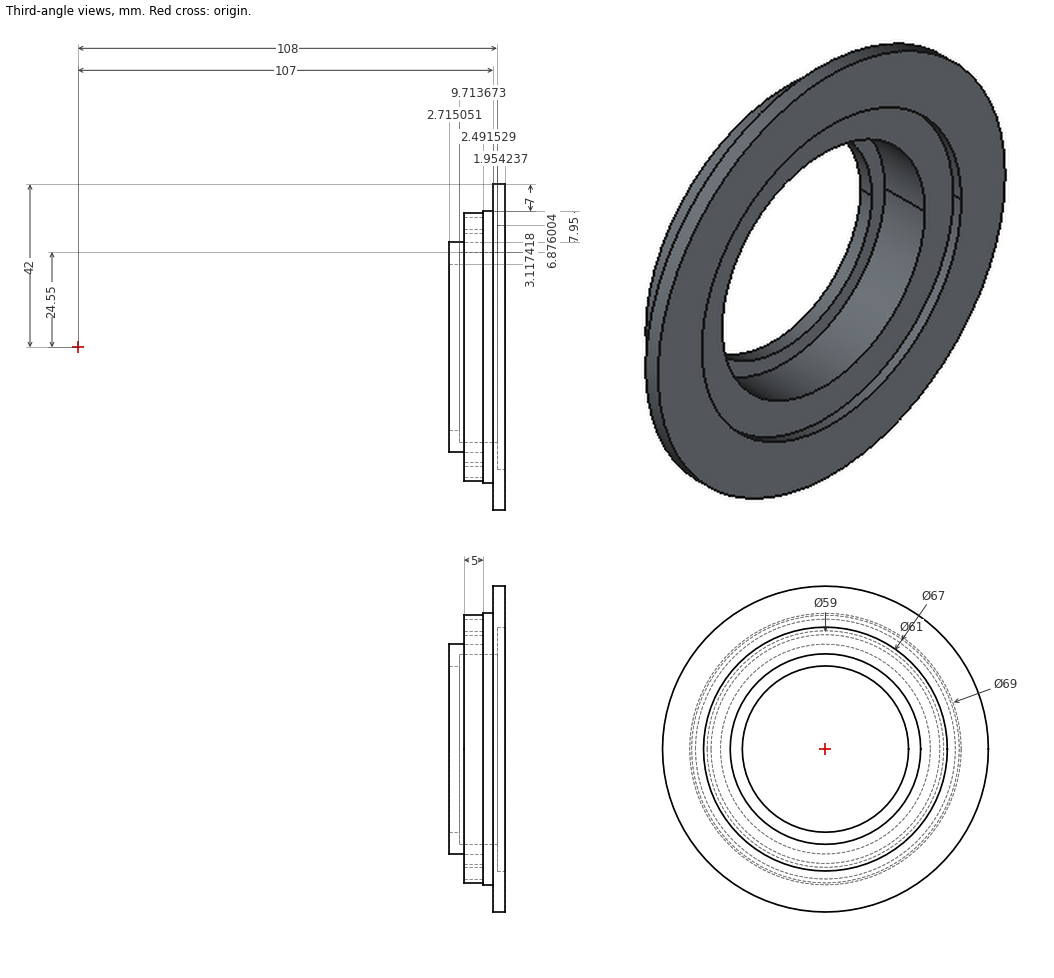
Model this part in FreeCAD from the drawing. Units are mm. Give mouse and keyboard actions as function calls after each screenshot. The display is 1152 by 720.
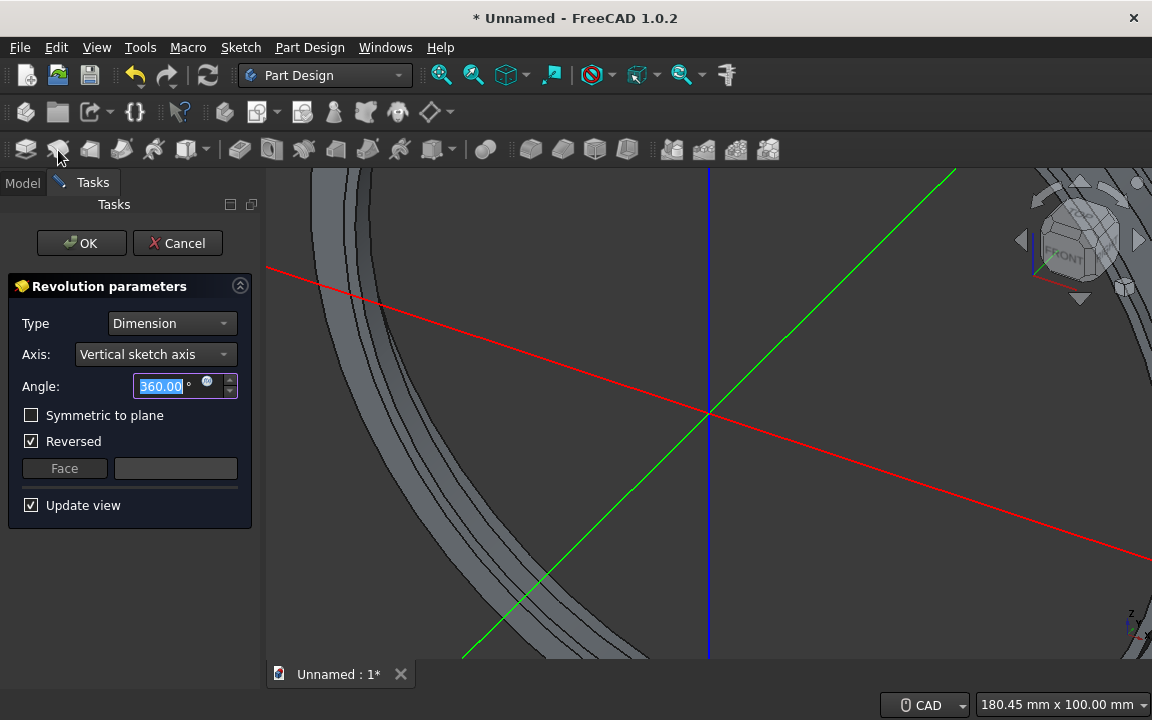
click(156, 354)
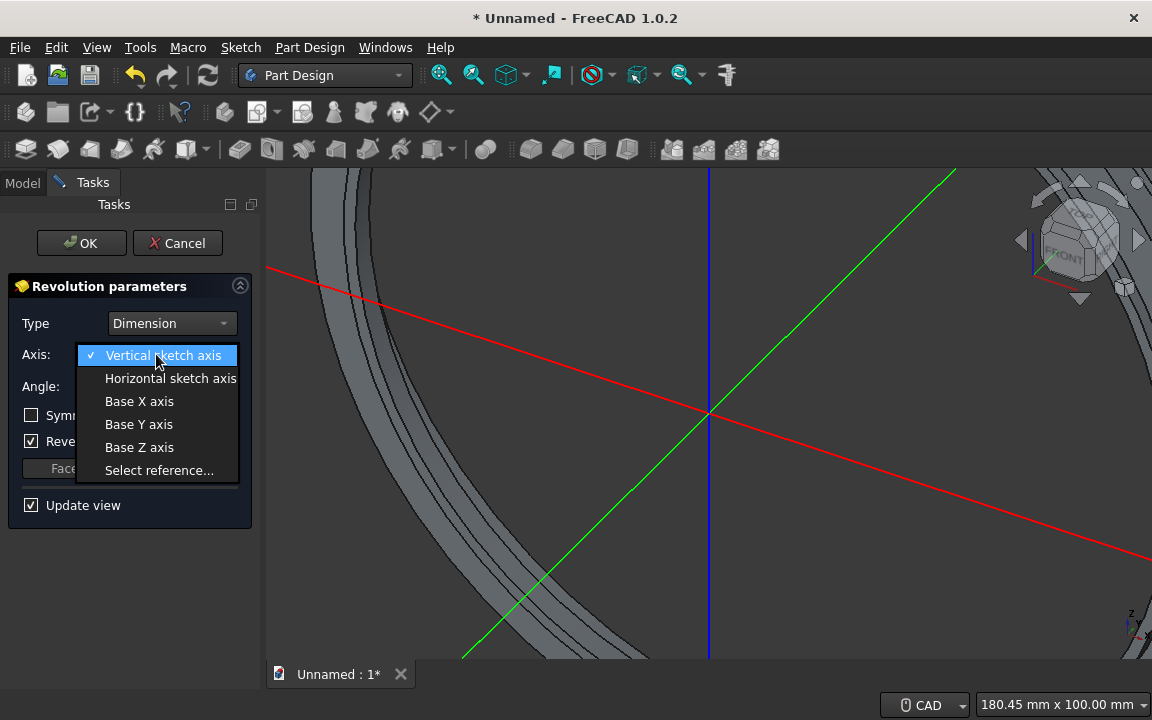
click(156, 378)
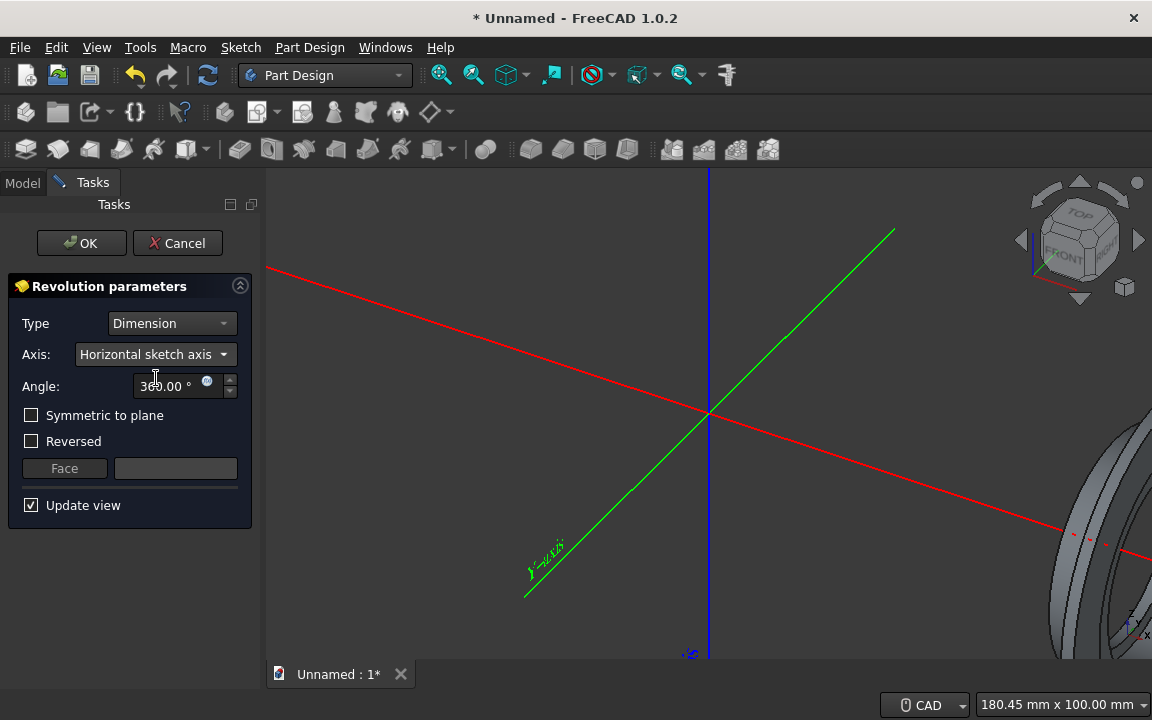
click(82, 243)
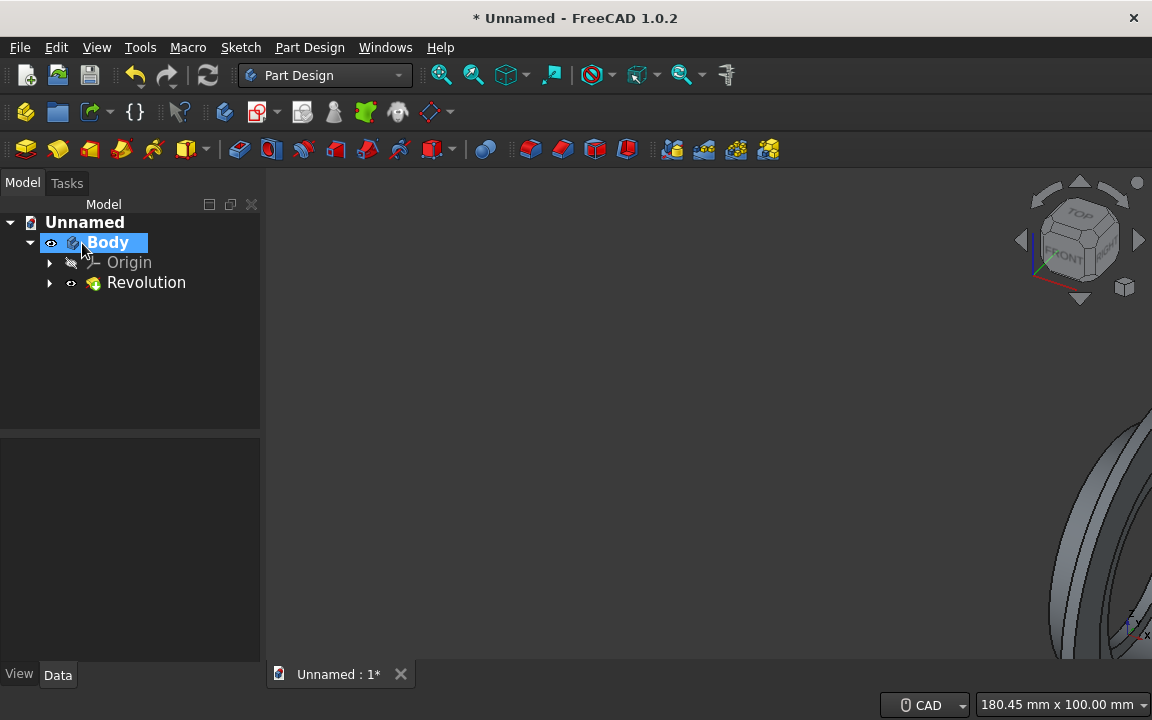
click(442, 76)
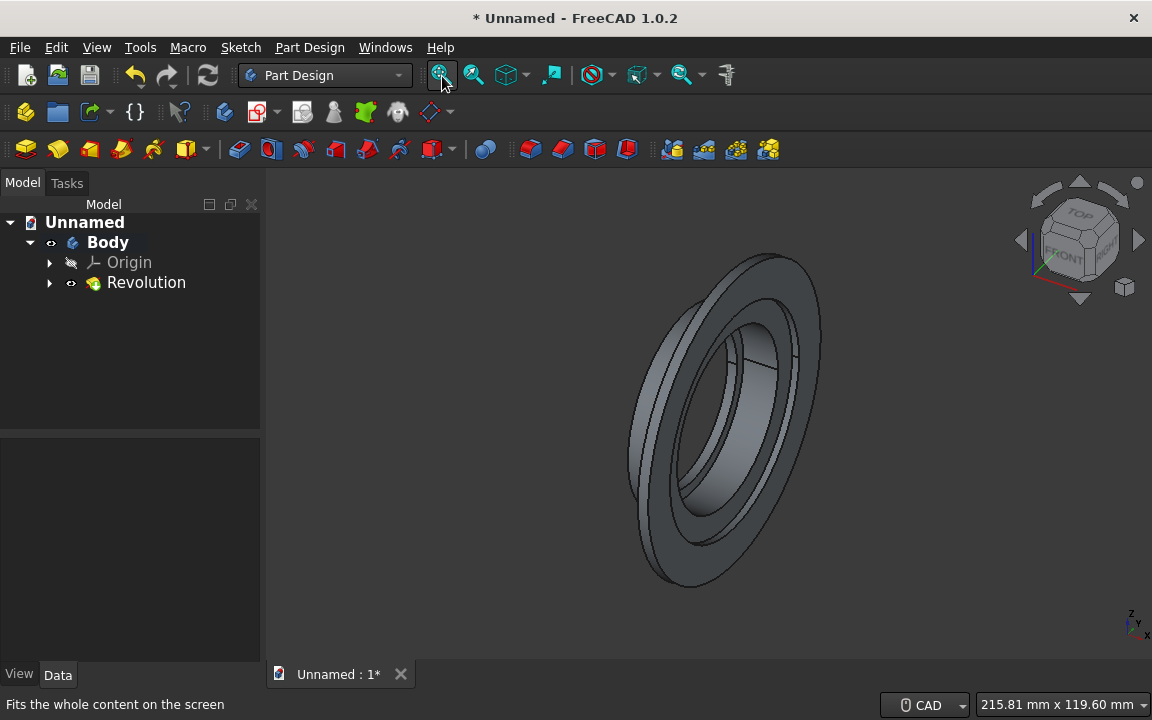
key(6)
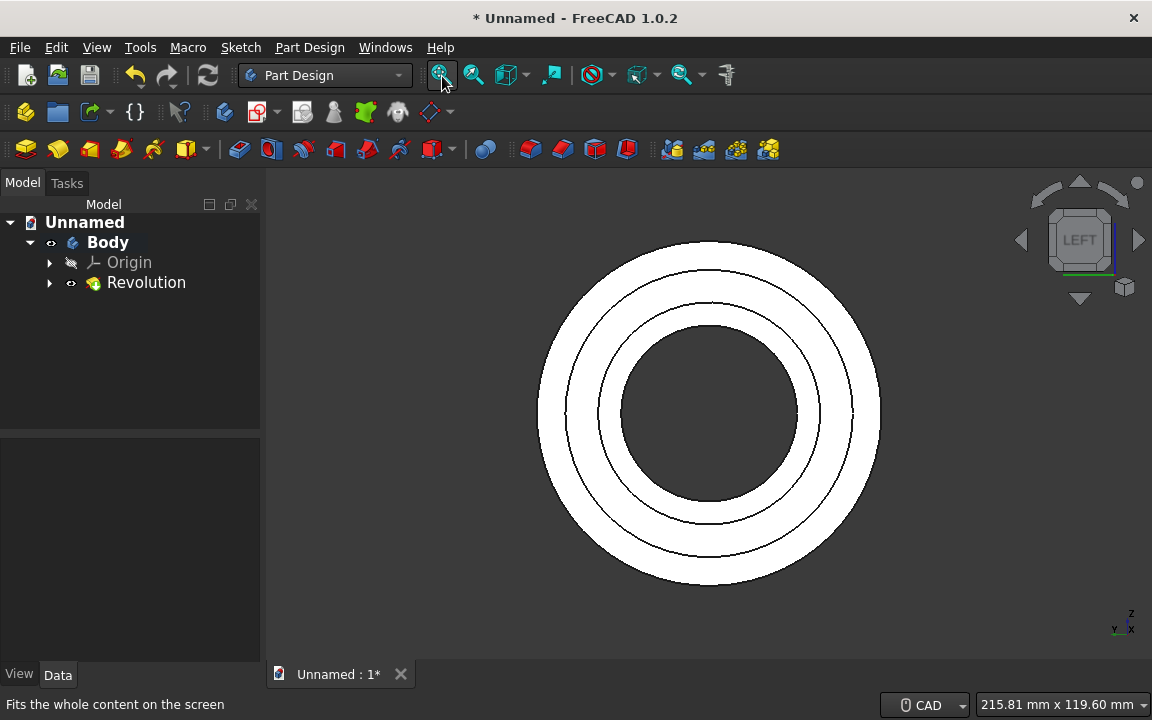
click(832, 454)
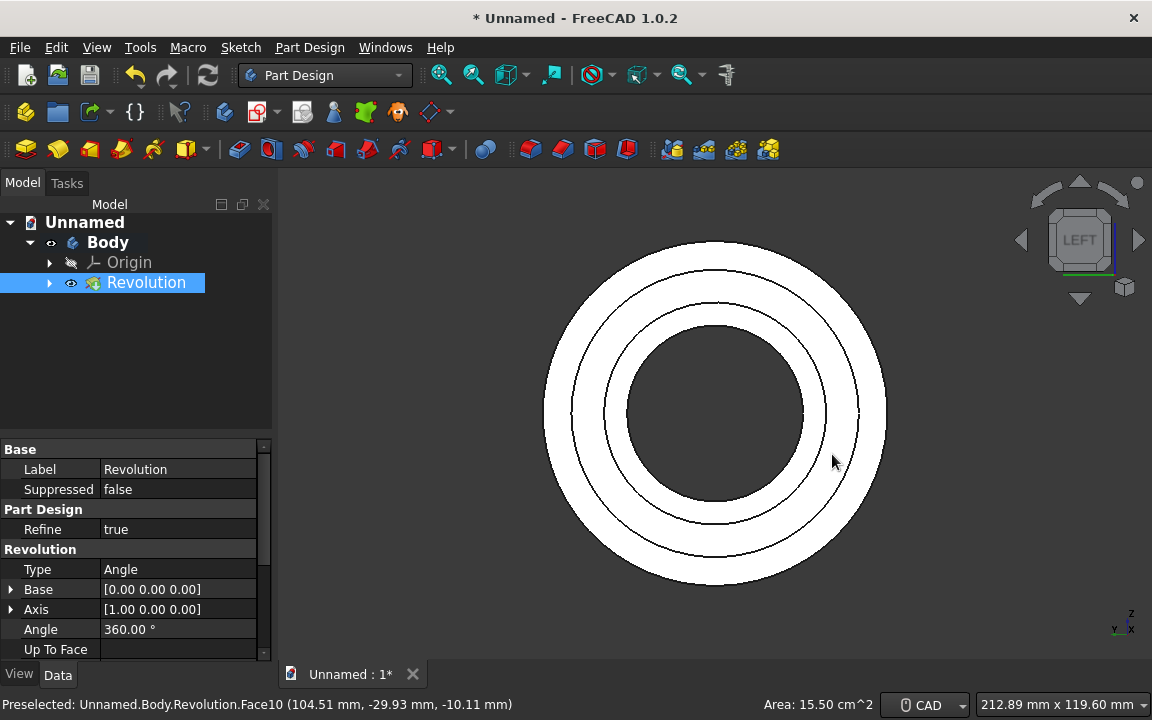
click(258, 112)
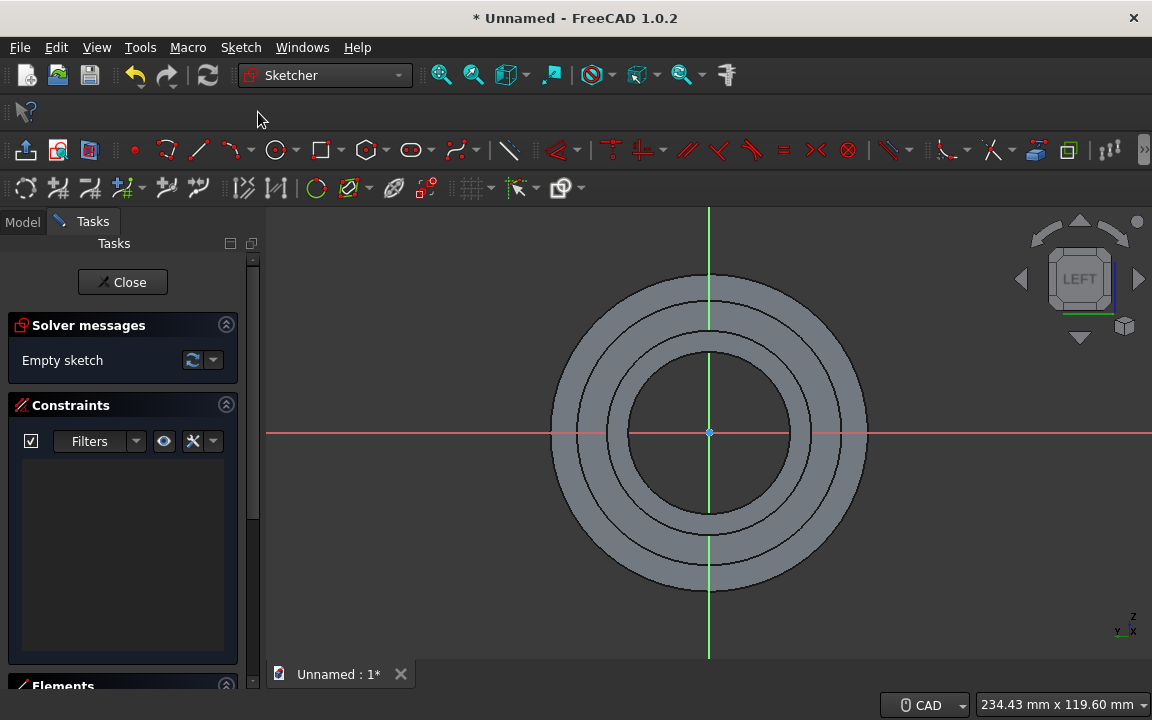
key(g)
key(c)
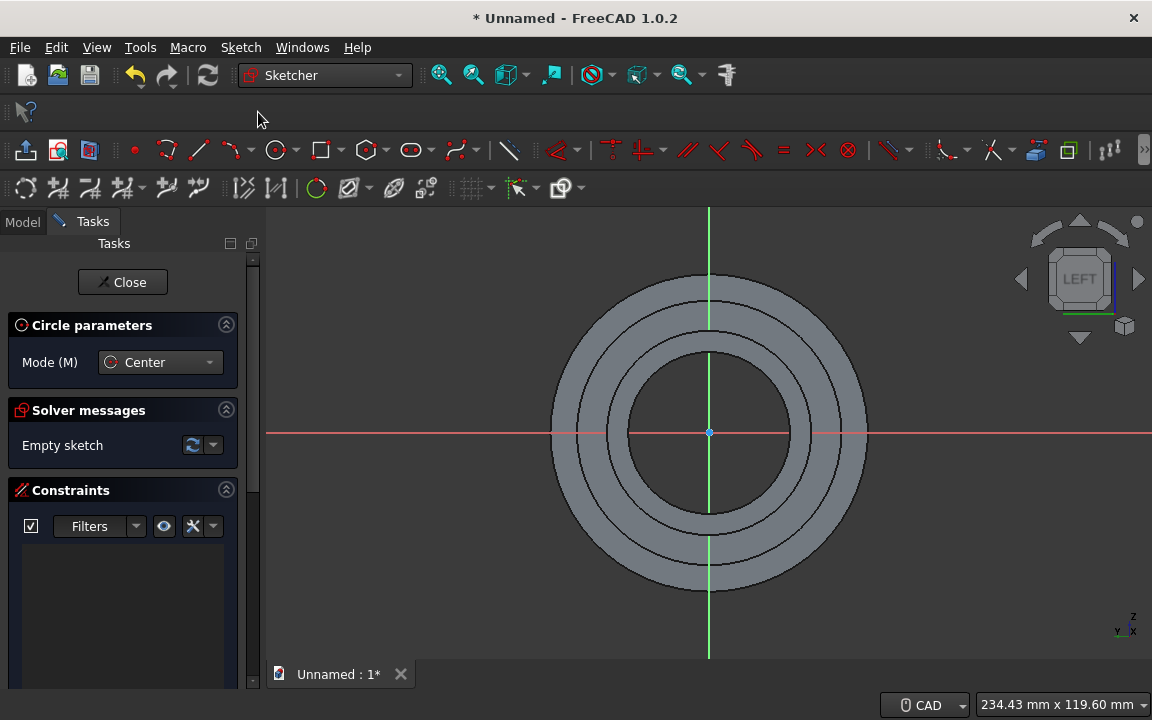
click(709, 433)
click(801, 341)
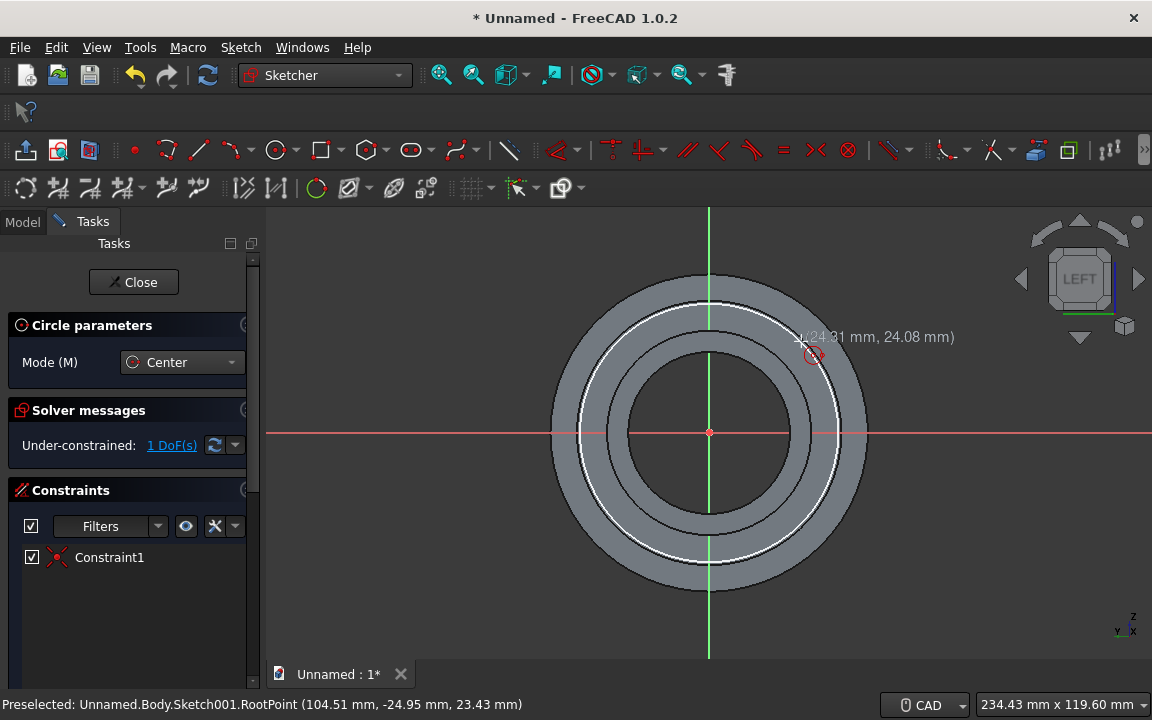
click(709, 433)
click(791, 351)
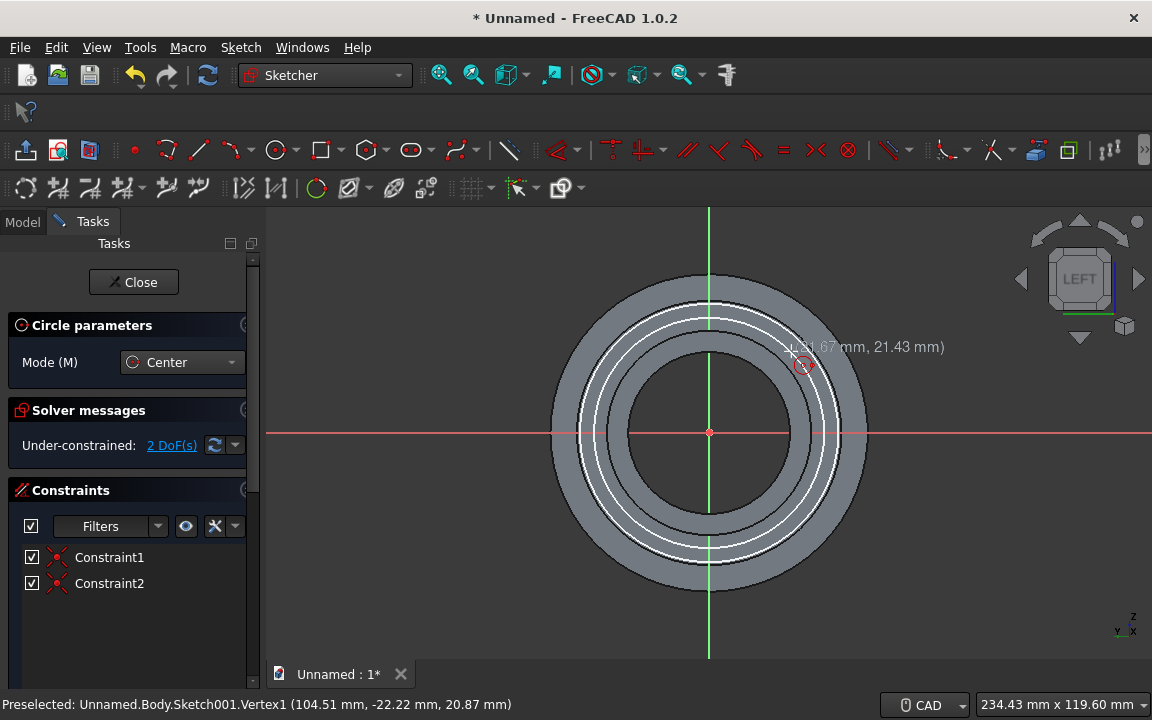
click(709, 433)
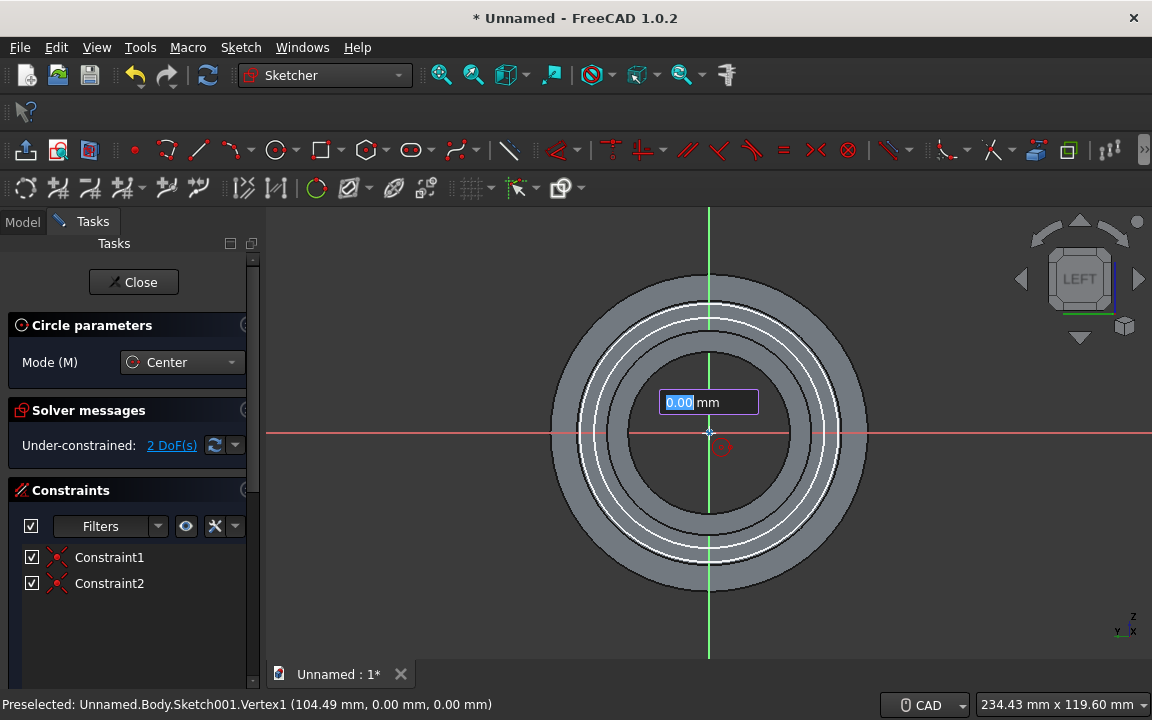
scroll(799, 343, up, 8)